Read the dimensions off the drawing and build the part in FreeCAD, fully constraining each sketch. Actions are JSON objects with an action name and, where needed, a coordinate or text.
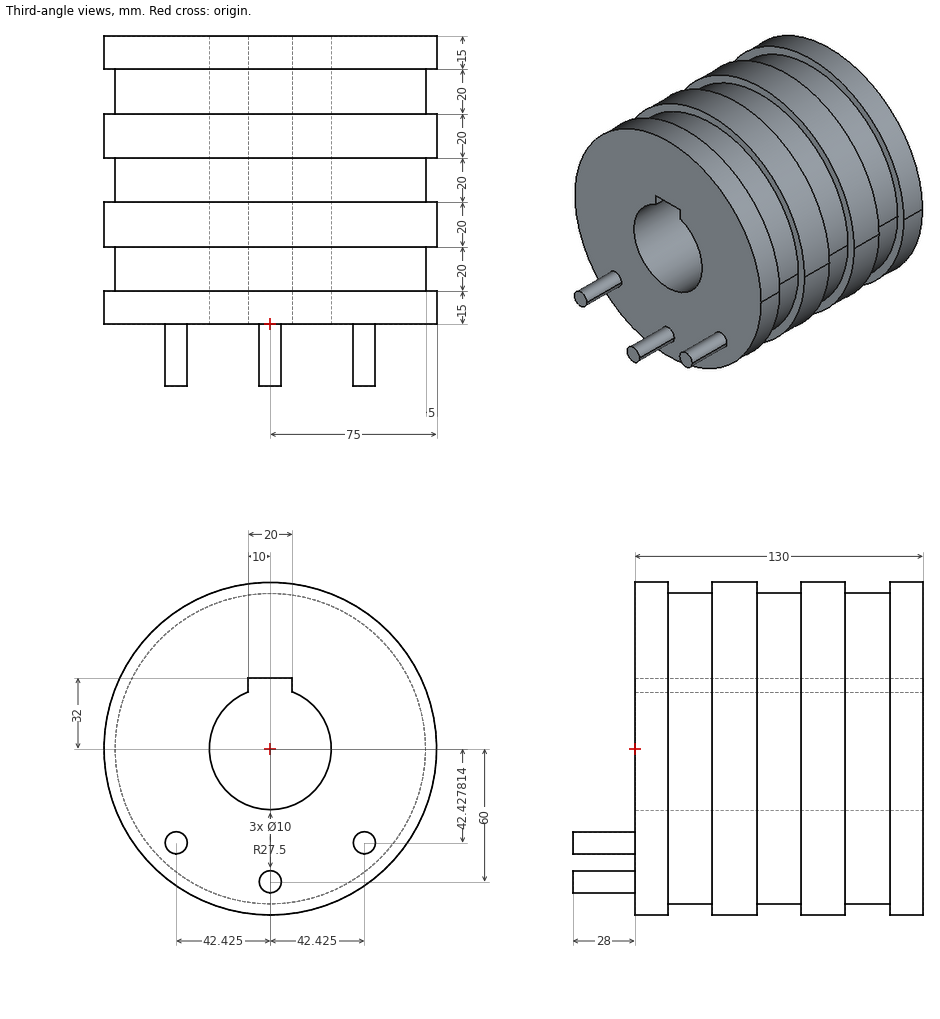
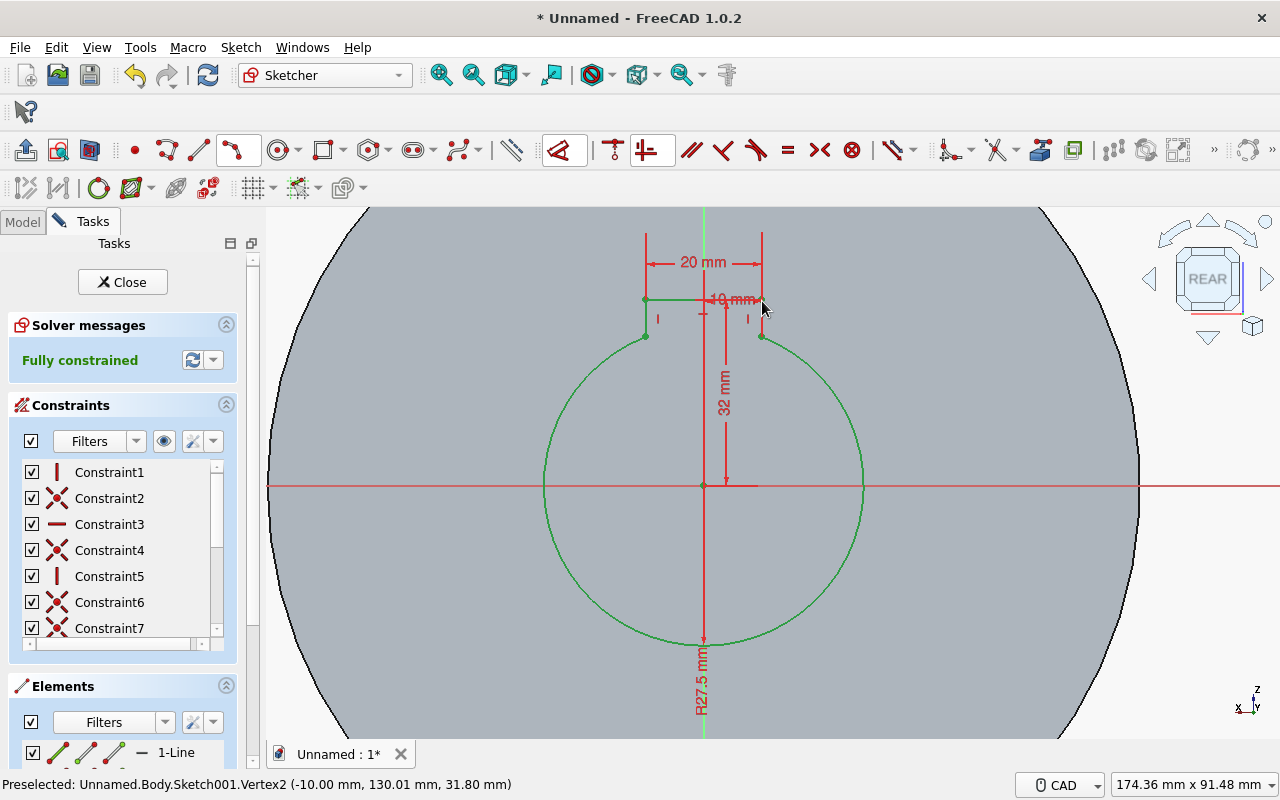
{"action": "left_click", "coordinate": [123, 282]}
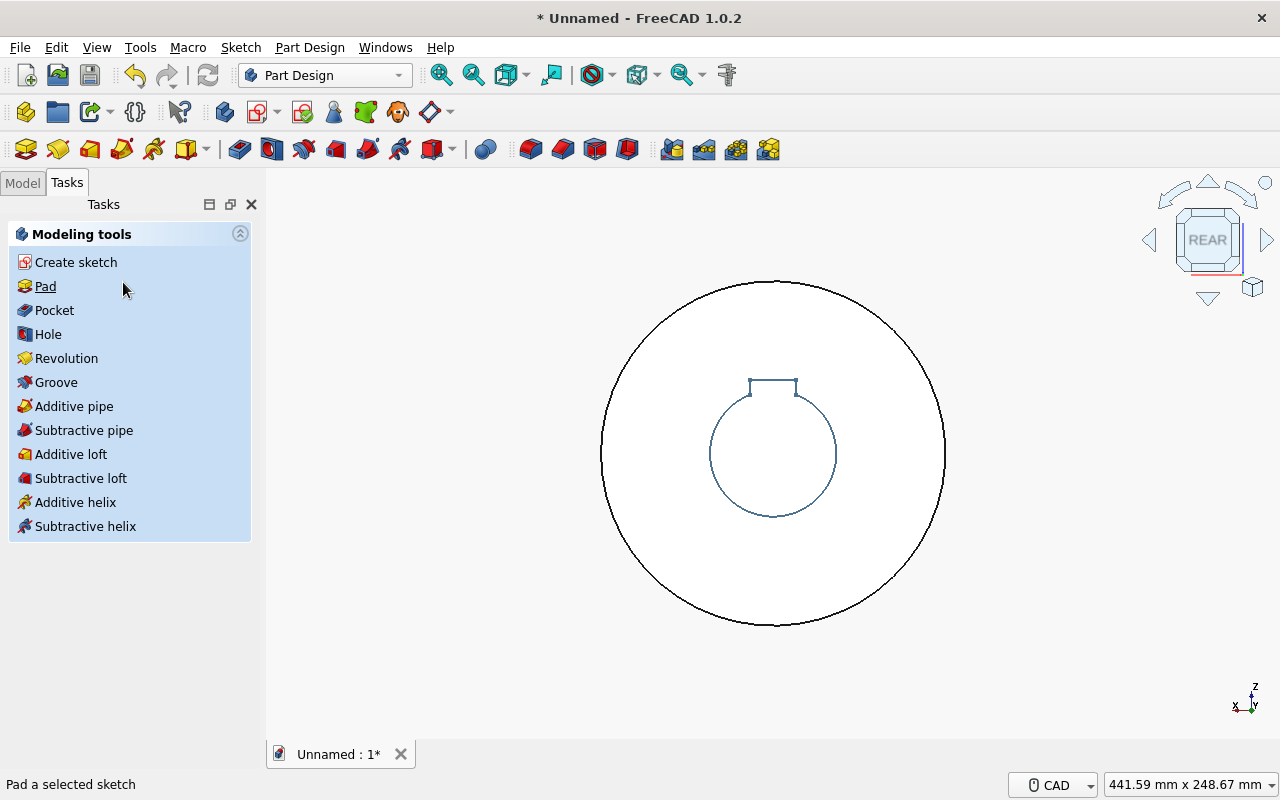
{"action": "left_click", "coordinate": [240, 150]}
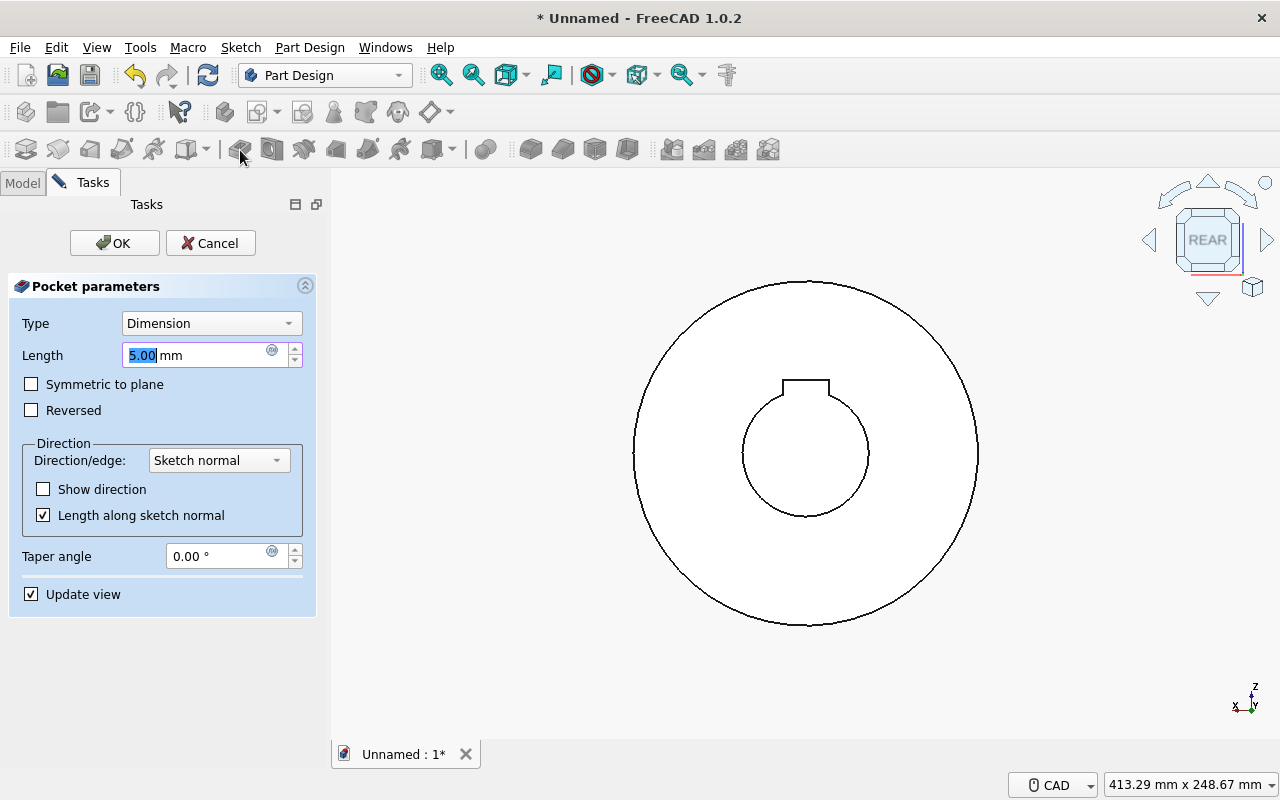
{"action": "type", "text": "130"}
{"action": "key", "text": "Tab"}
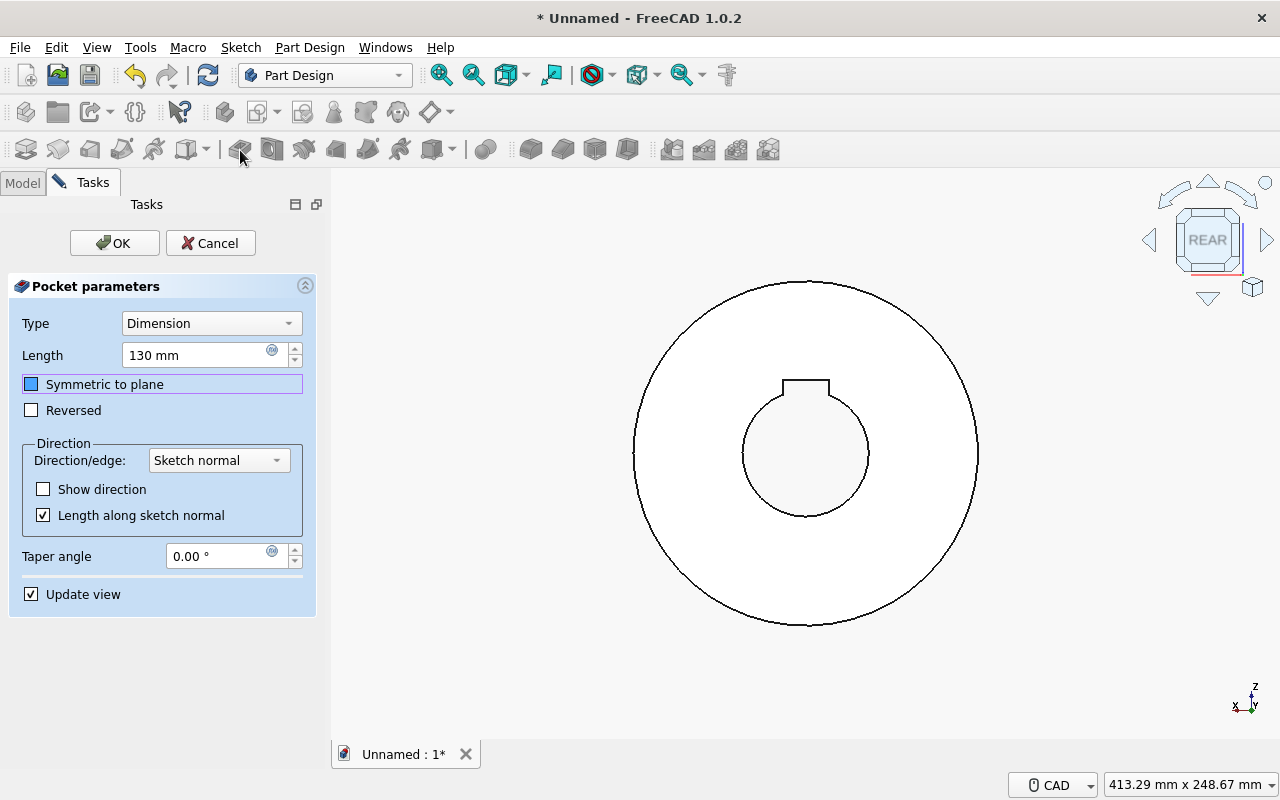
{"action": "left_click", "coordinate": [115, 243]}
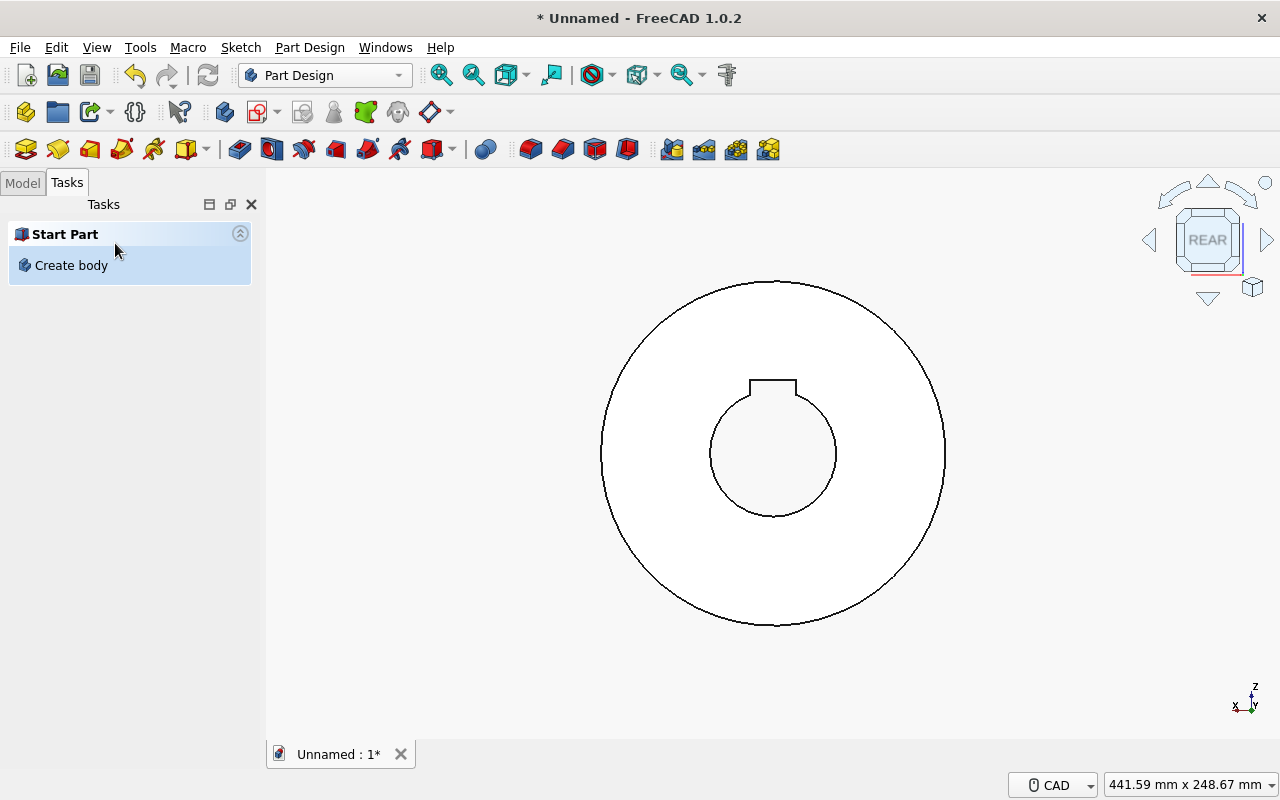
{"action": "key", "text": "0"}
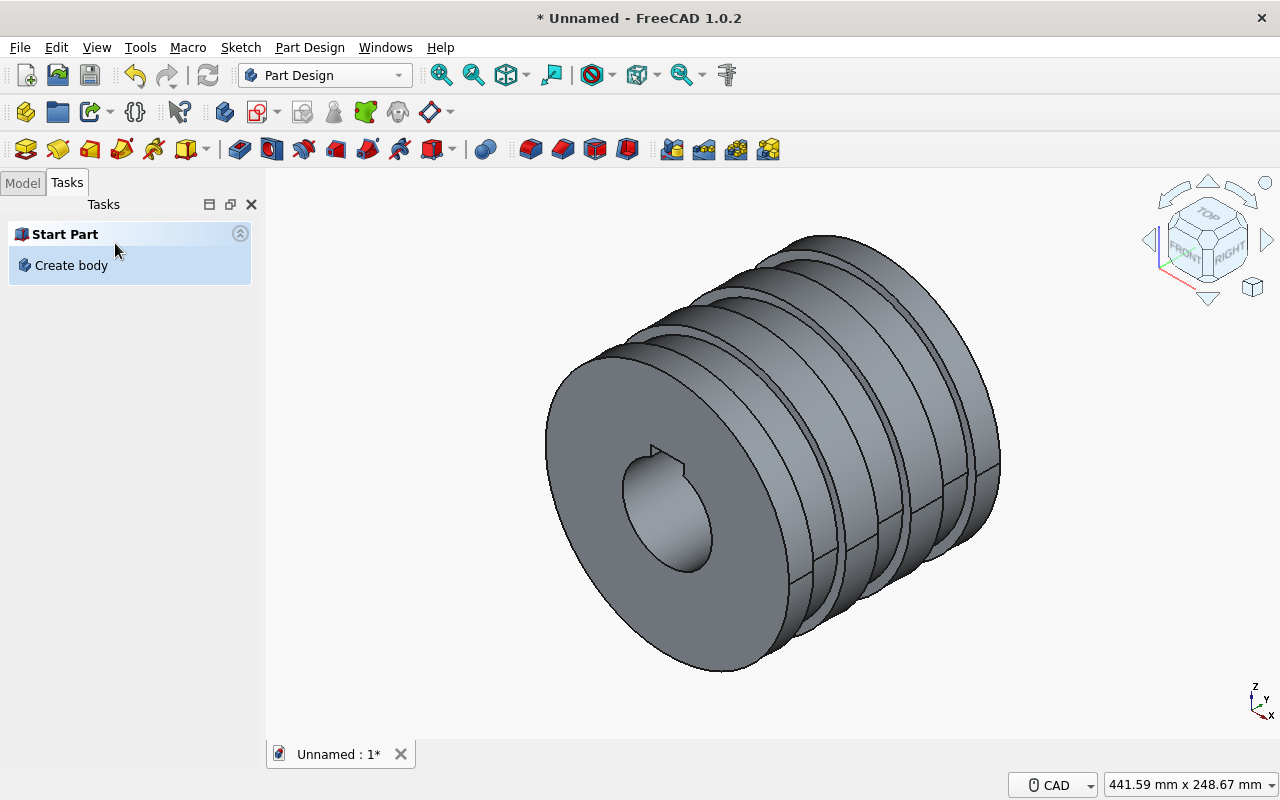
{"action": "left_click", "coordinate": [702, 614]}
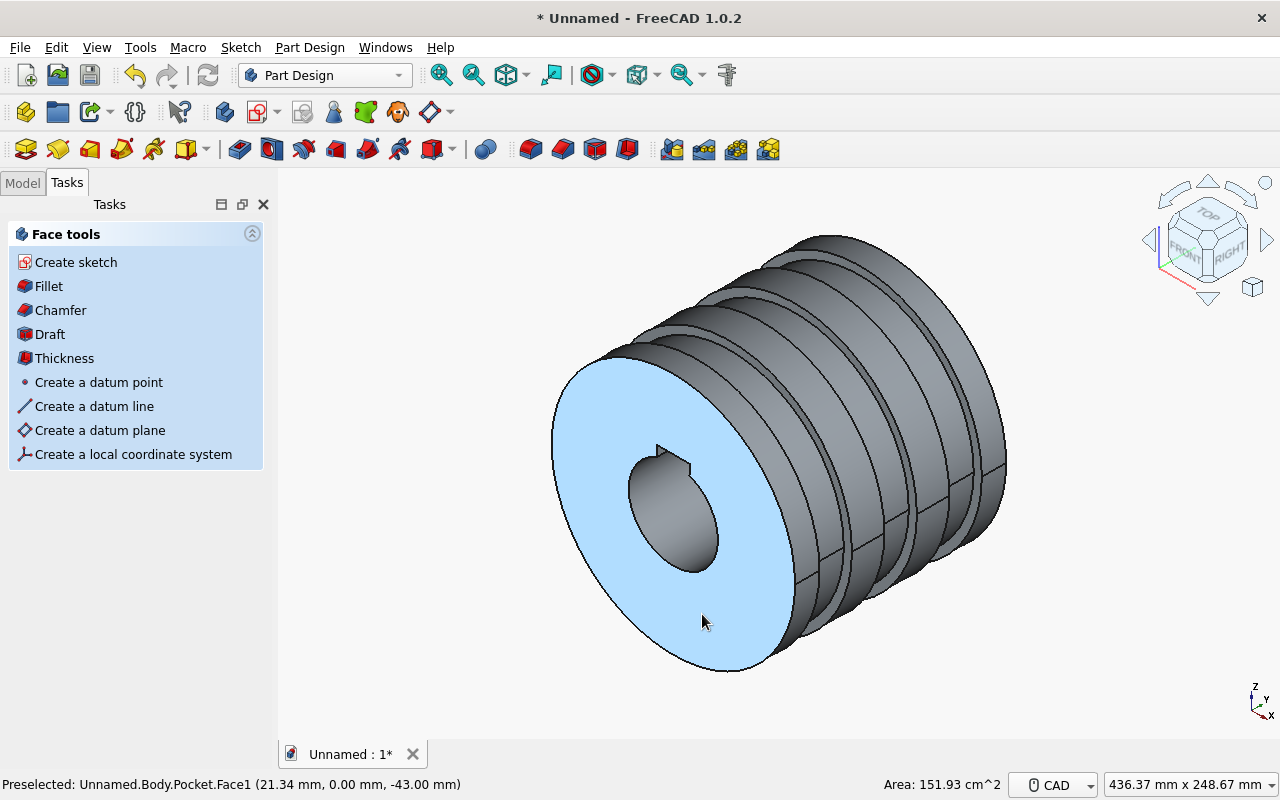
{"action": "left_click", "coordinate": [258, 112]}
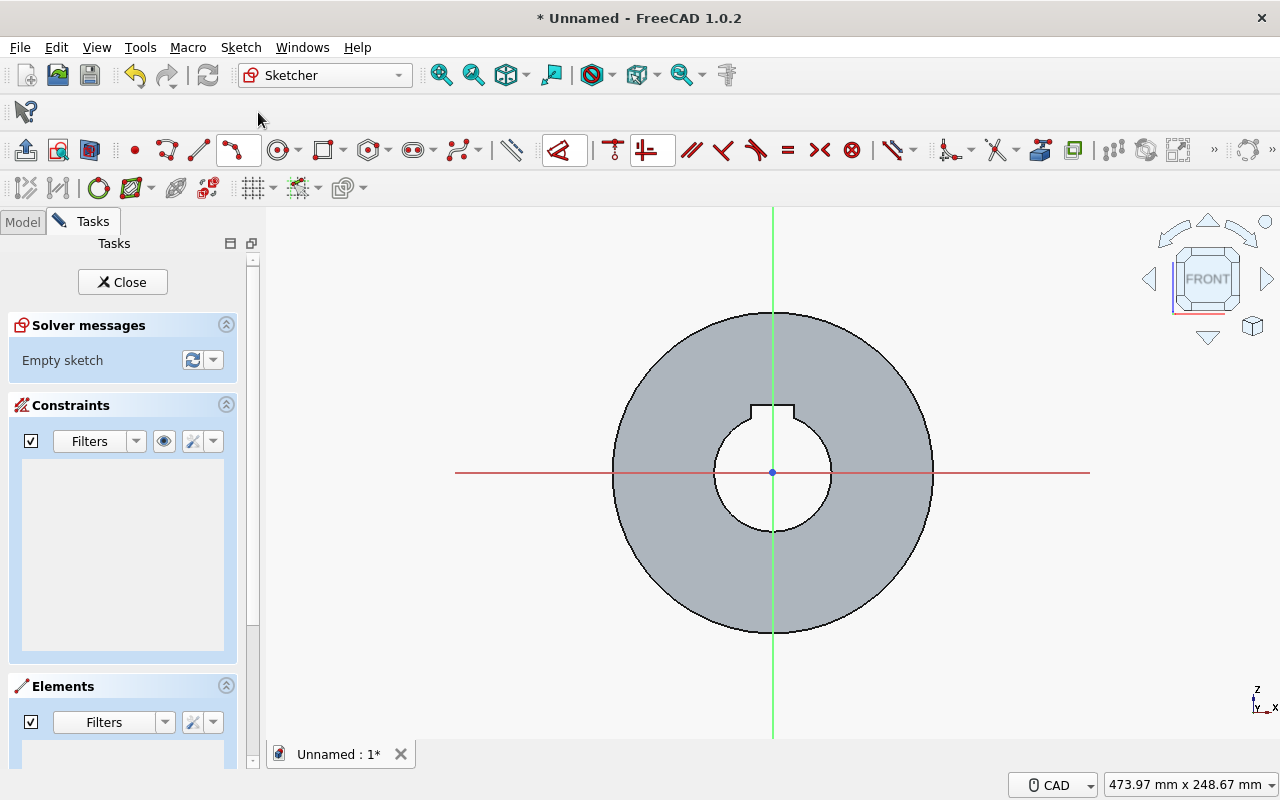
{"action": "scroll", "coordinate": [829, 599], "scroll_direction": "up", "scroll_amount": 4}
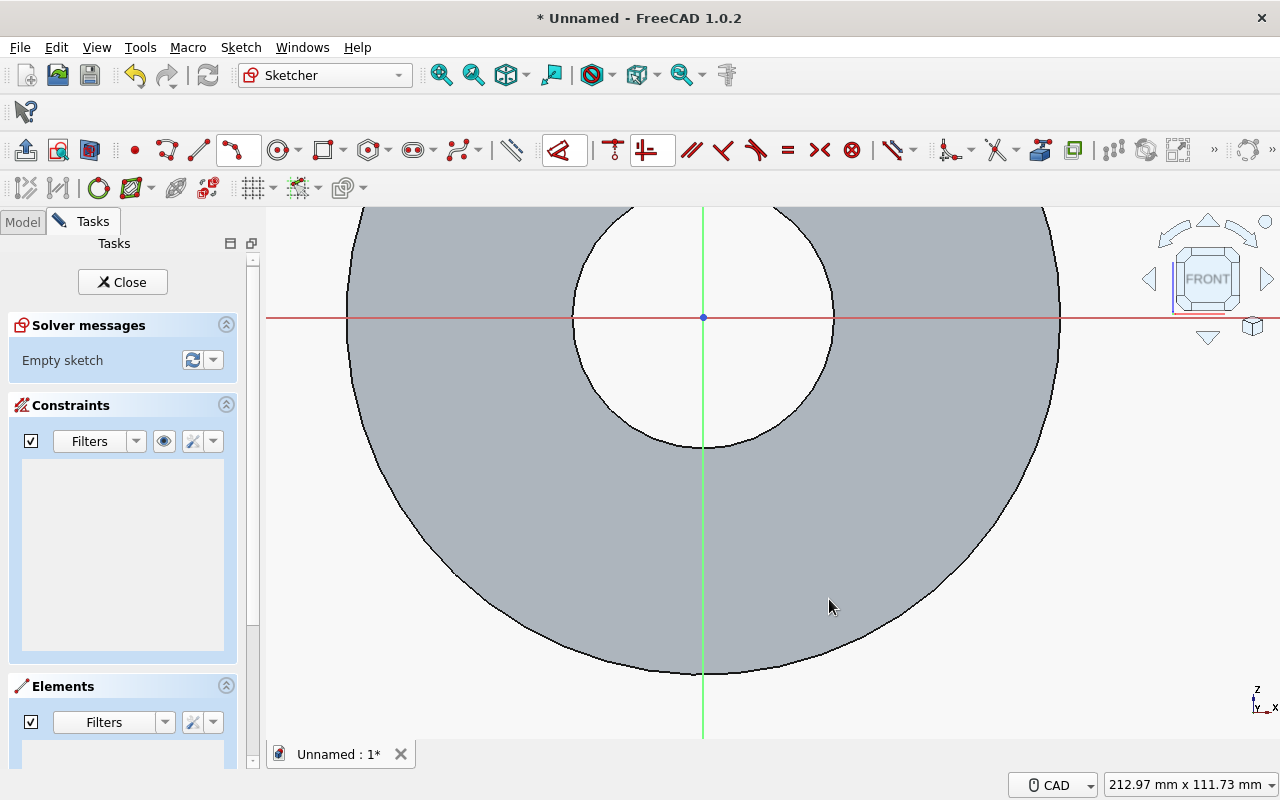
{"action": "left_click", "coordinate": [278, 150]}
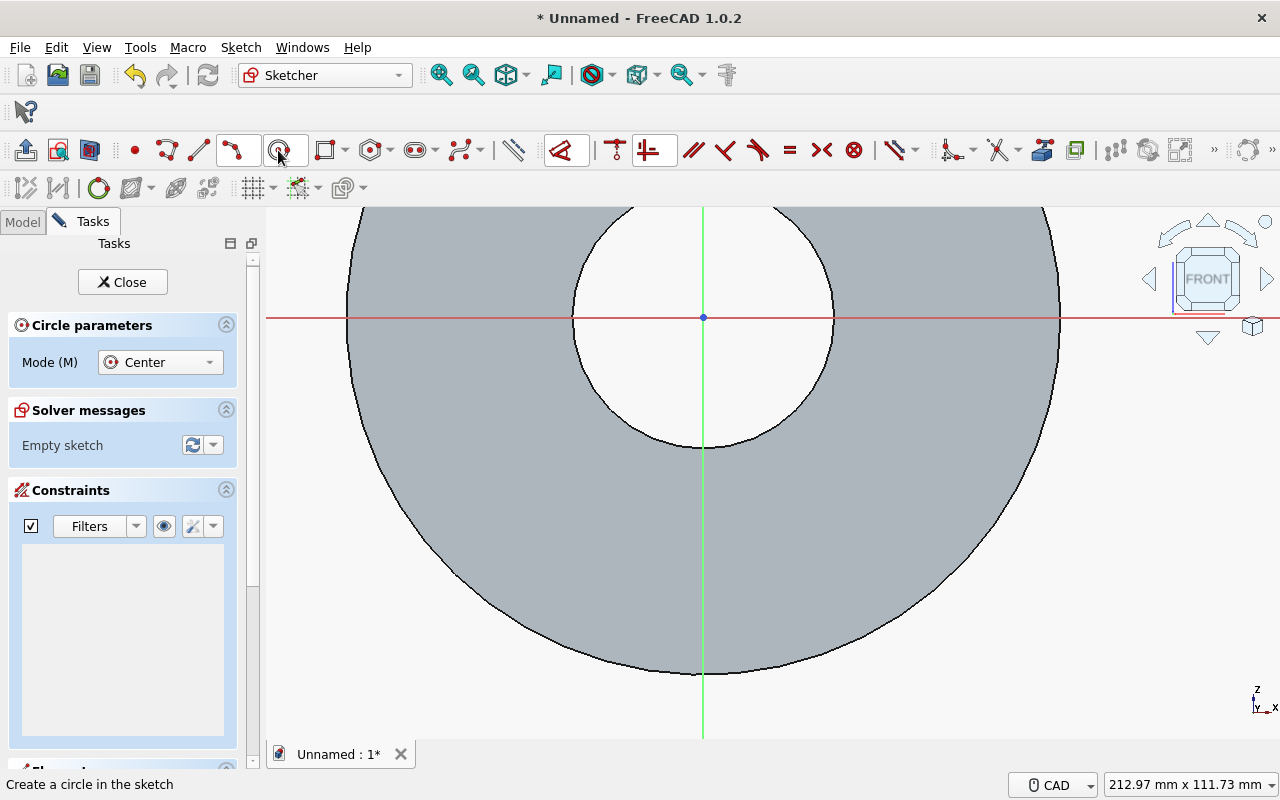
{"action": "left_click", "coordinate": [703, 603]}
{"action": "mouse_move", "coordinate": [720, 587]}